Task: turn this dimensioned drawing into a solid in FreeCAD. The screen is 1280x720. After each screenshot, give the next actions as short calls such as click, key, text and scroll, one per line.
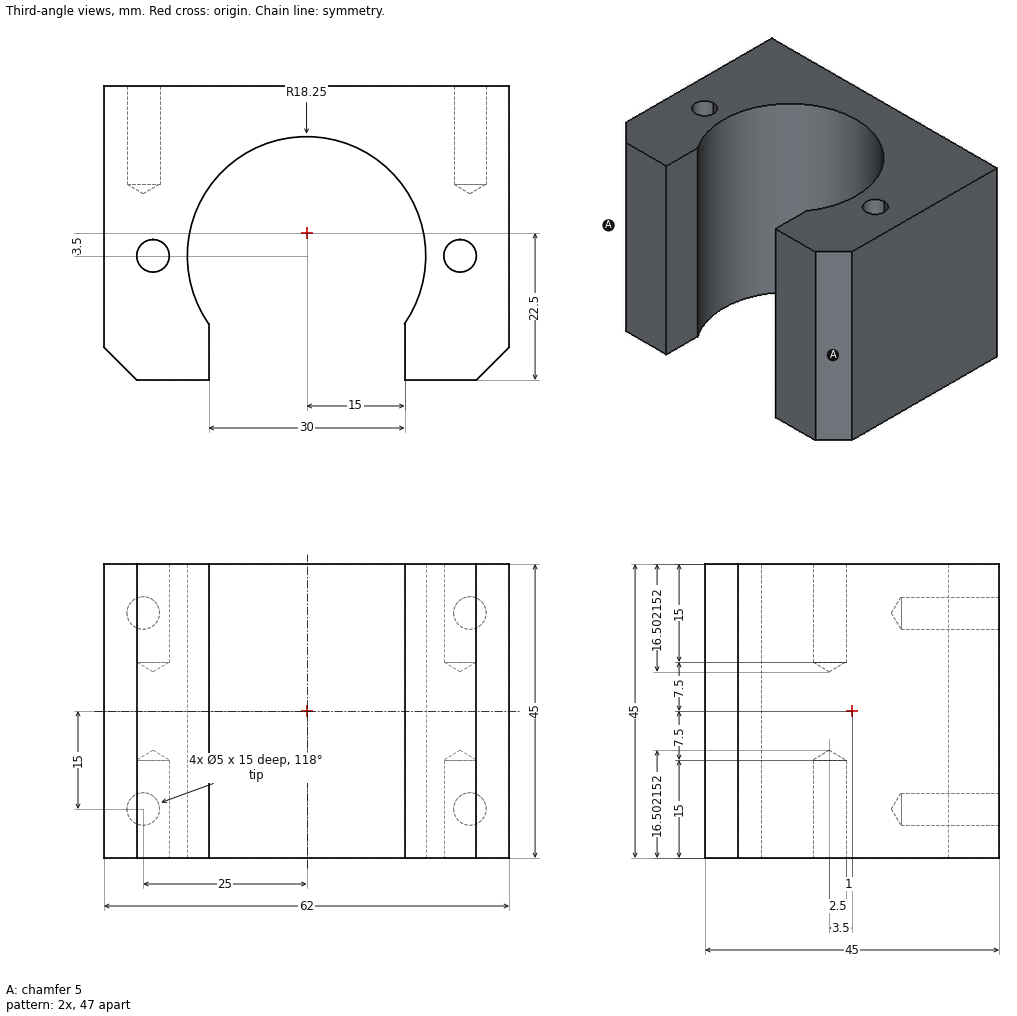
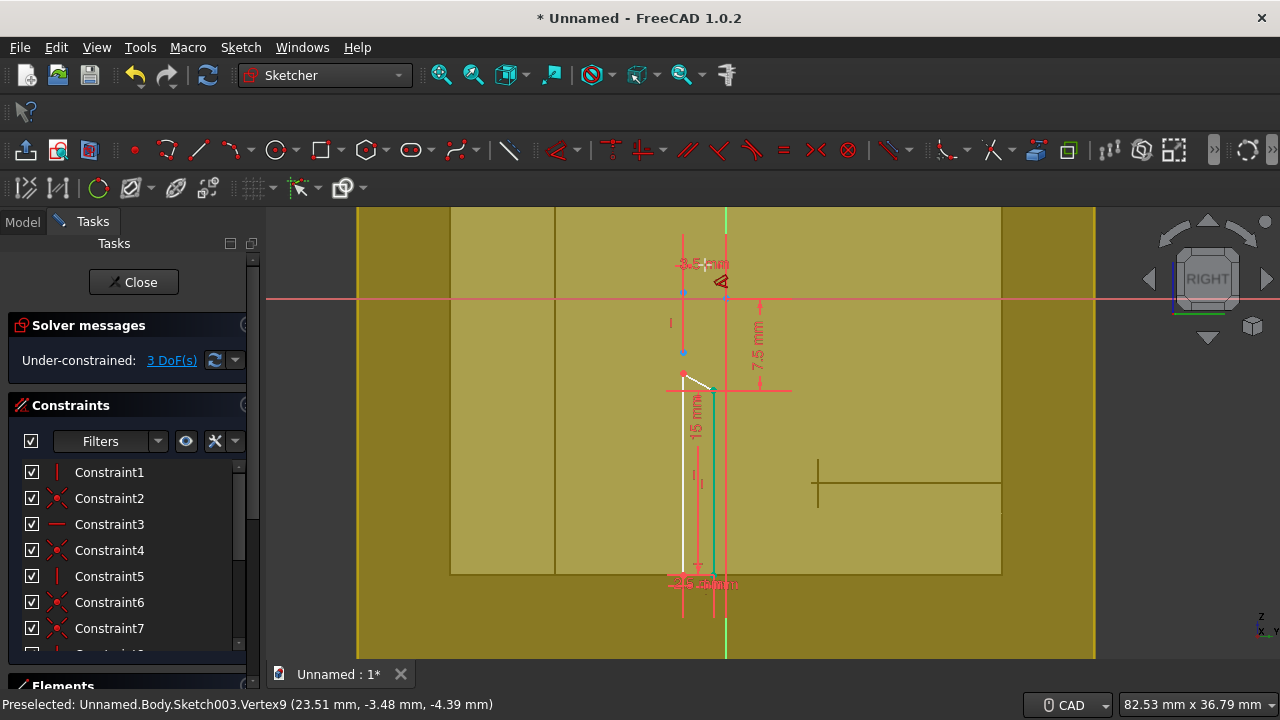
click(683, 434)
click(649, 475)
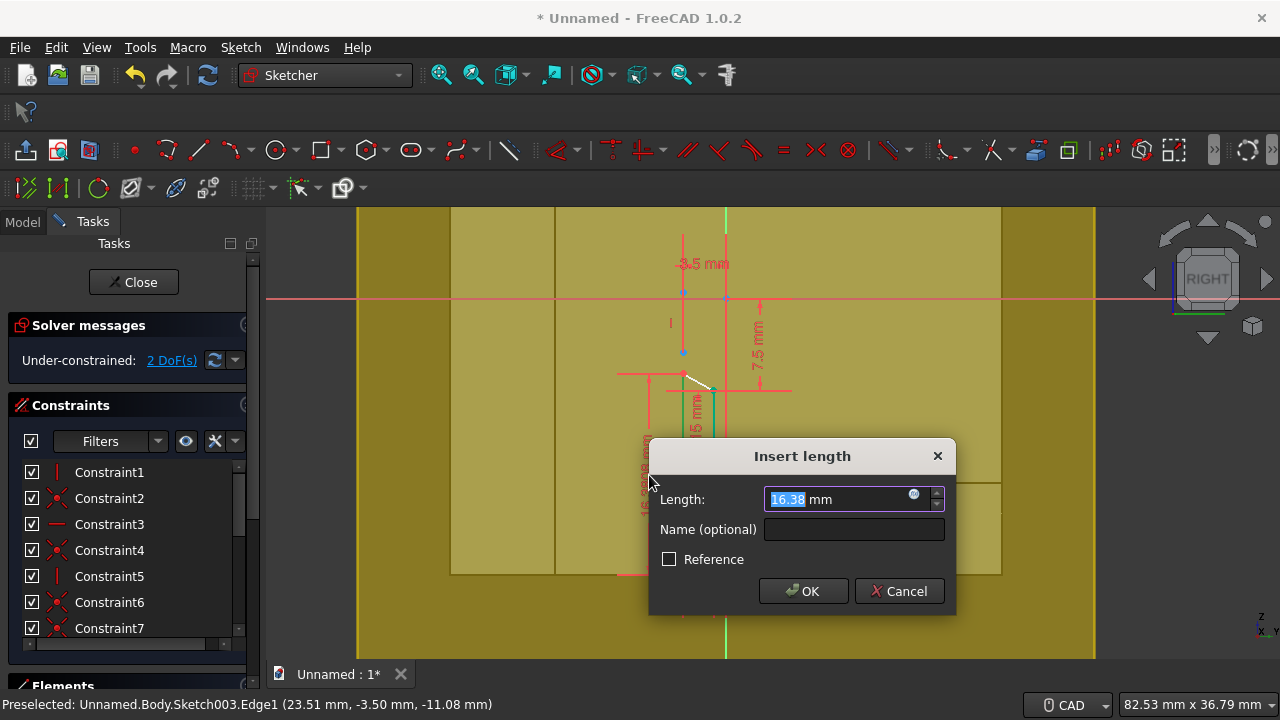
text(16.502152)
key(Return)
key(Escape)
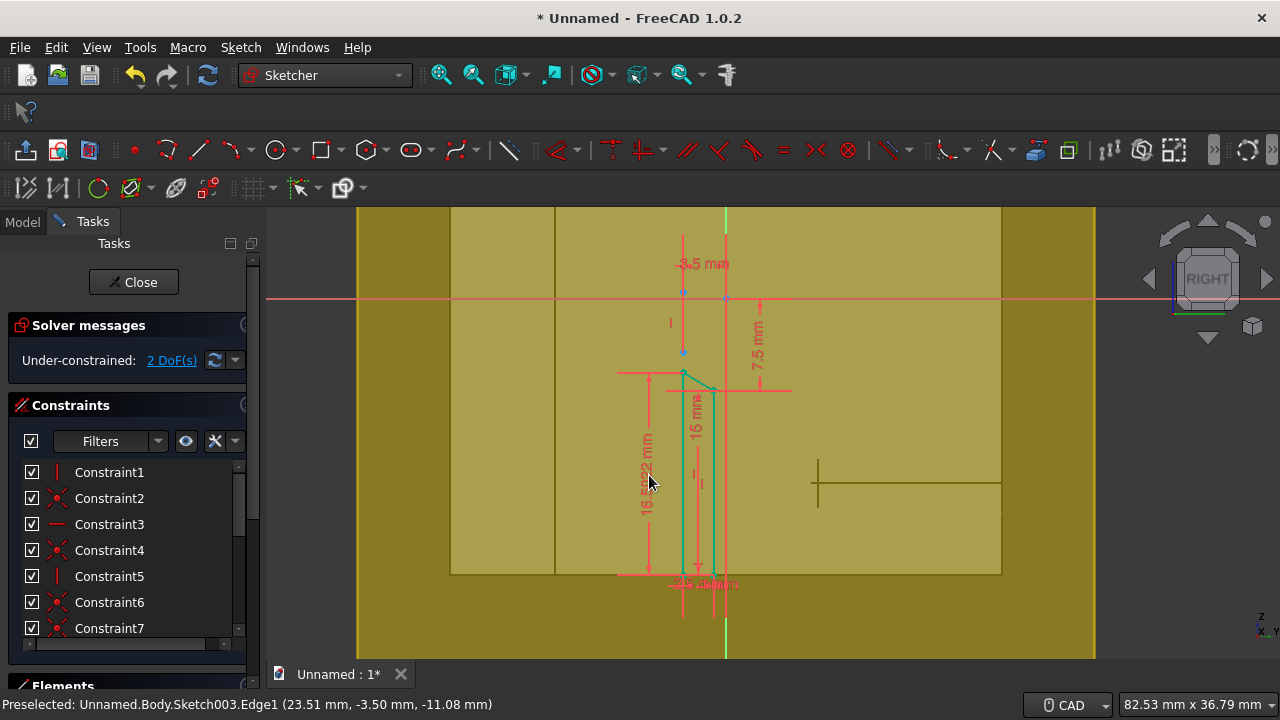
click(134, 282)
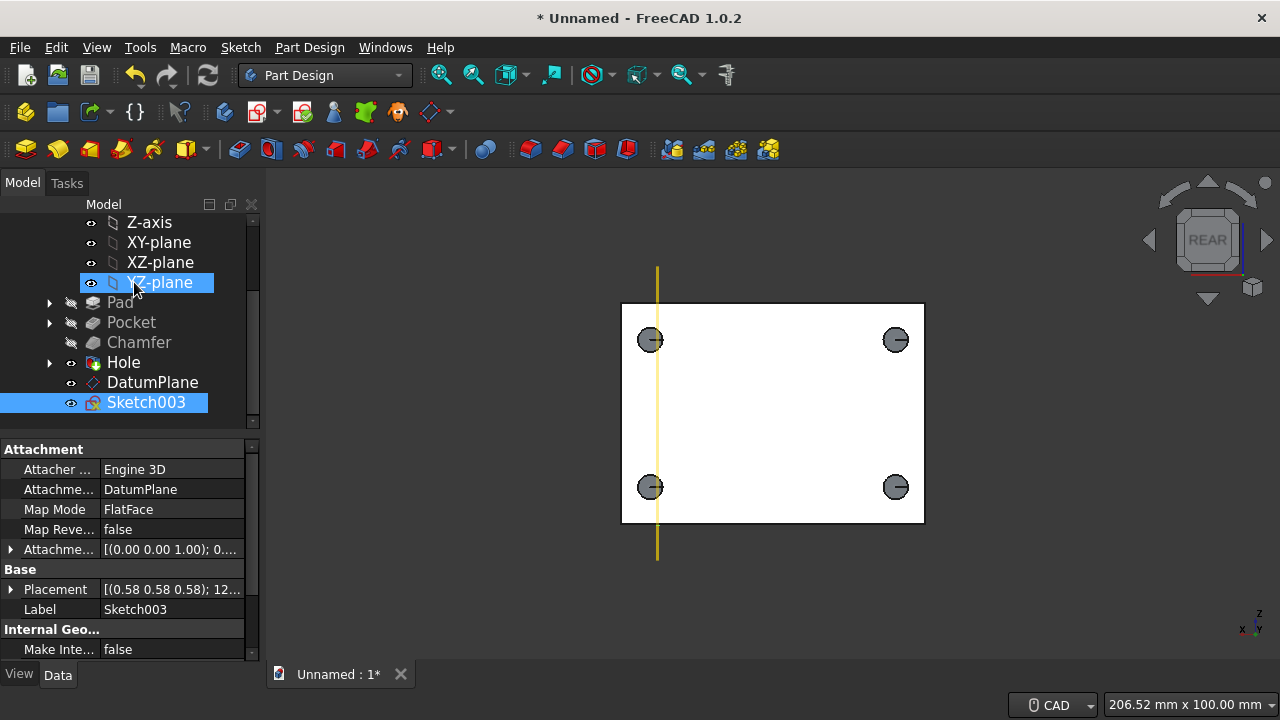
click(304, 150)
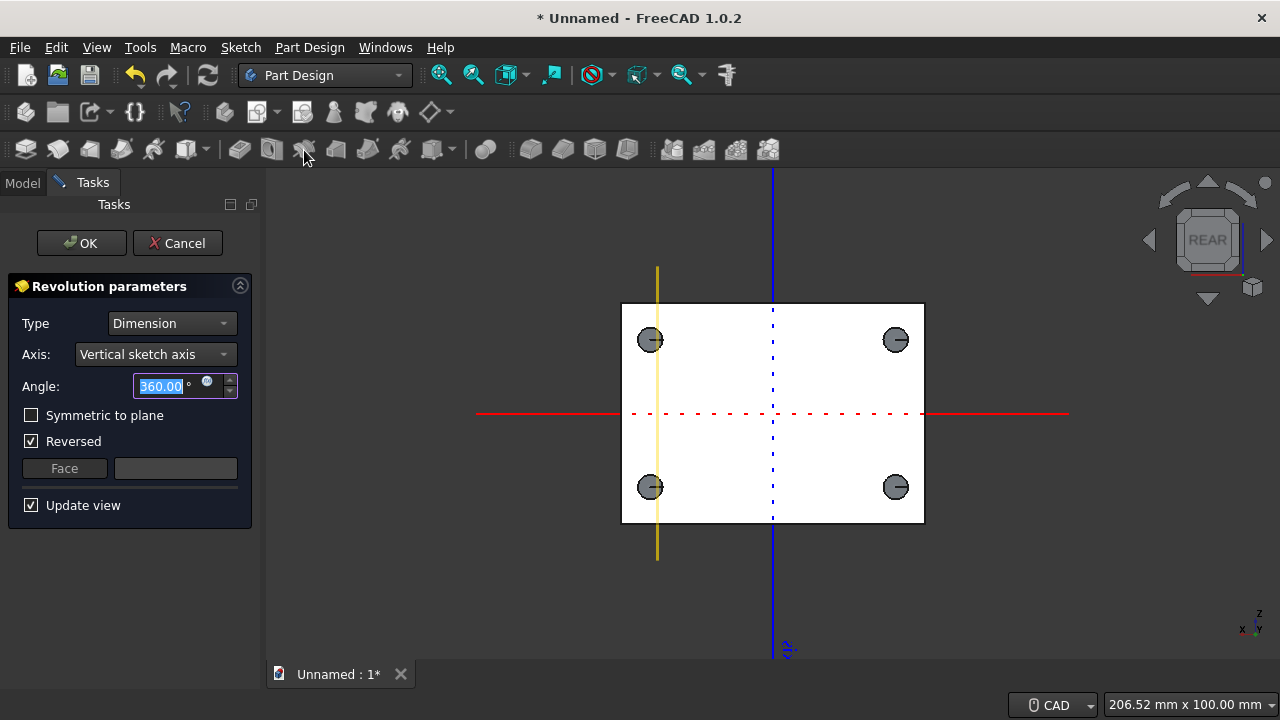
click(156, 354)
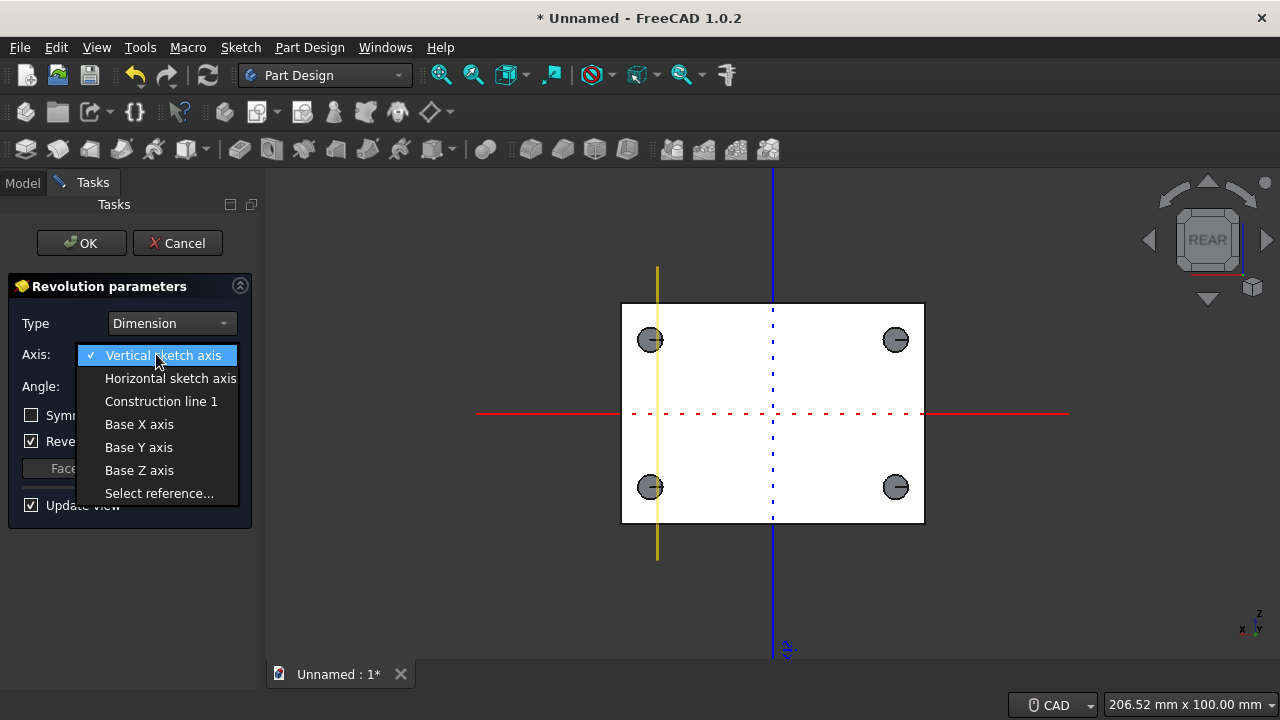
click(156, 402)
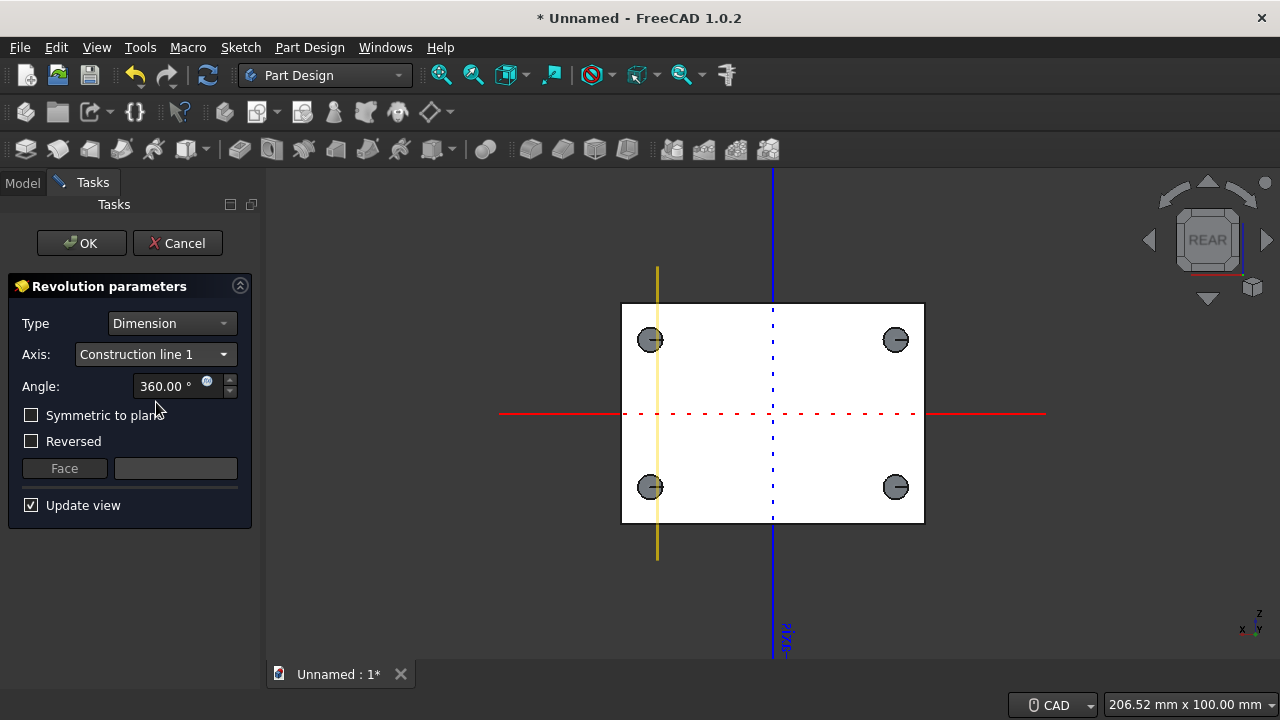
click(82, 243)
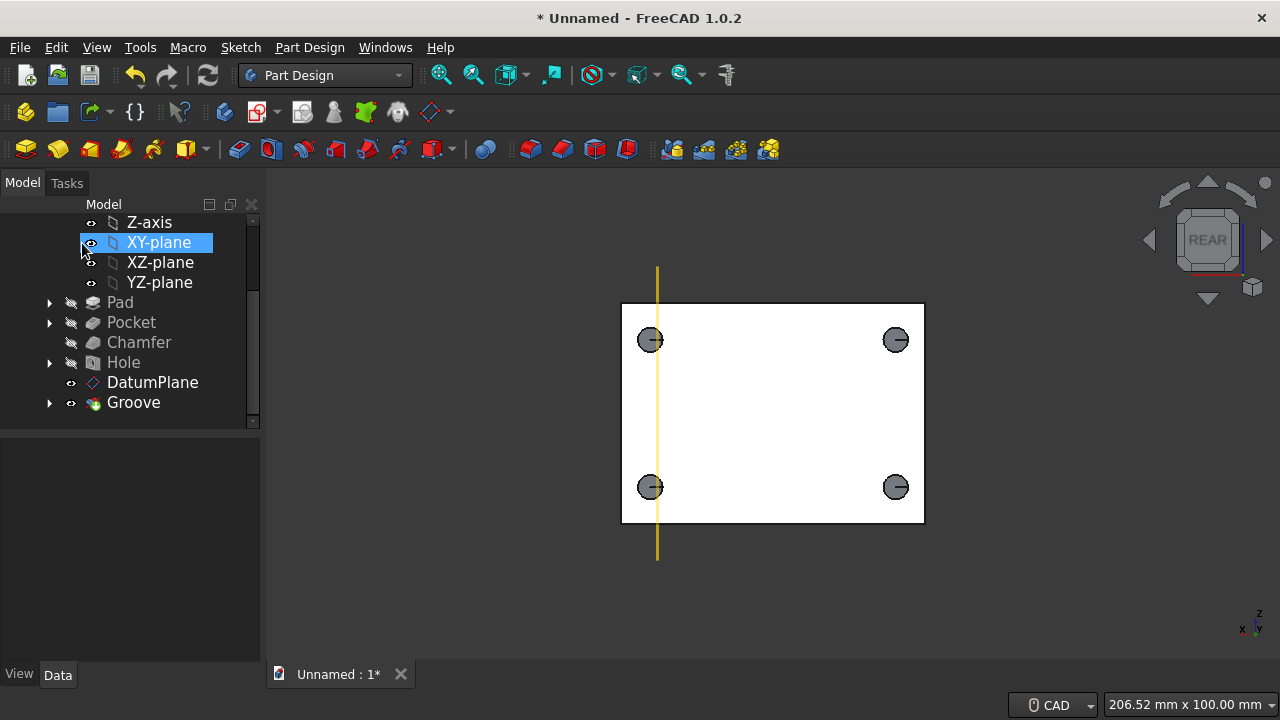
click(116, 383)
key(space)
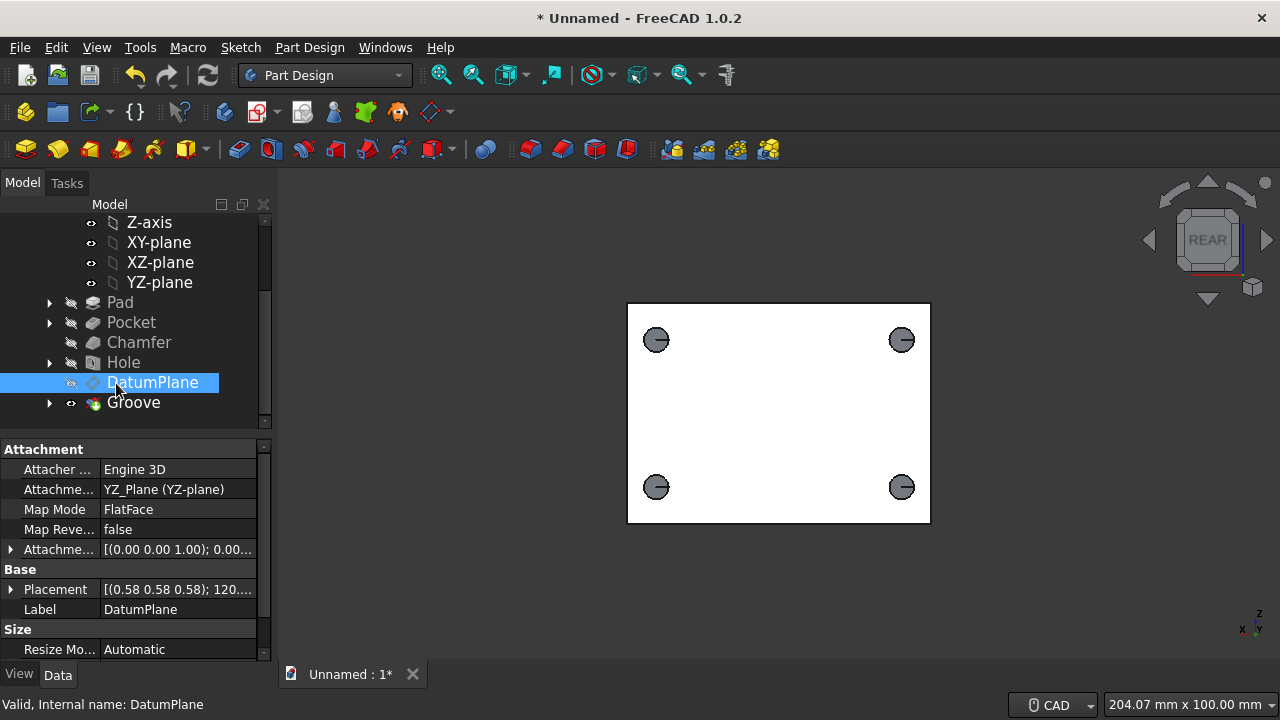
click(116, 403)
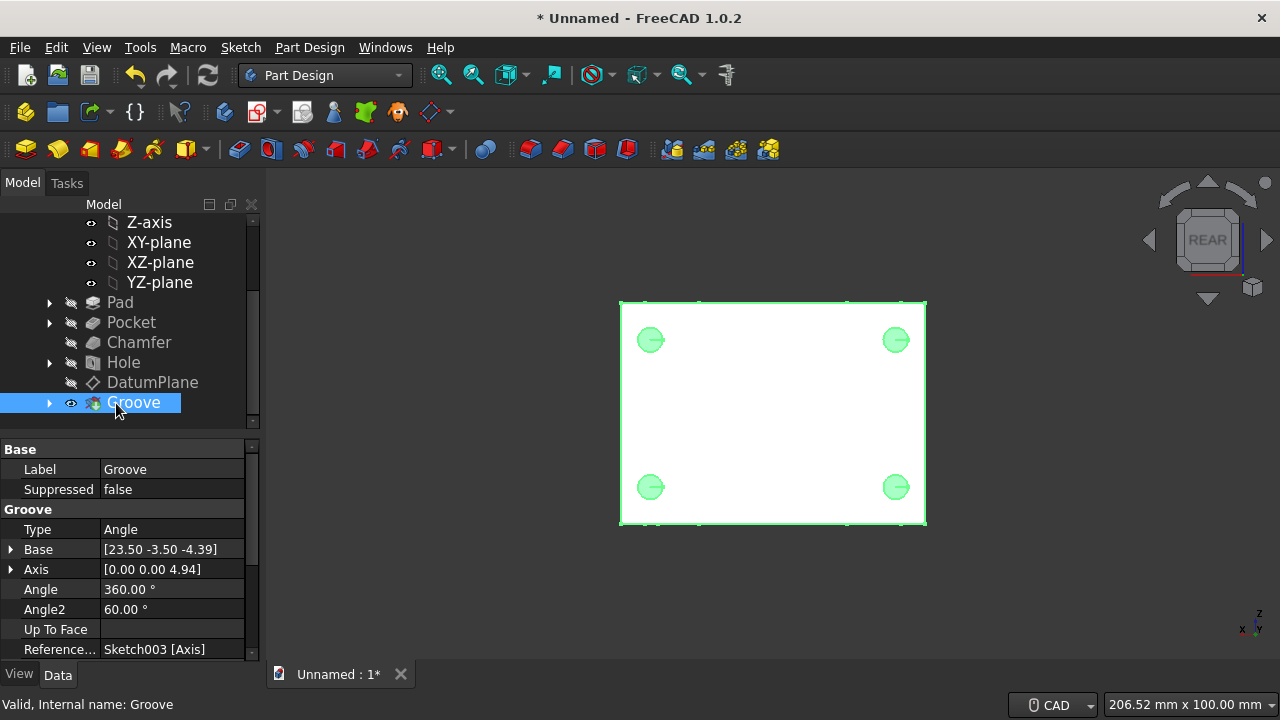
click(704, 150)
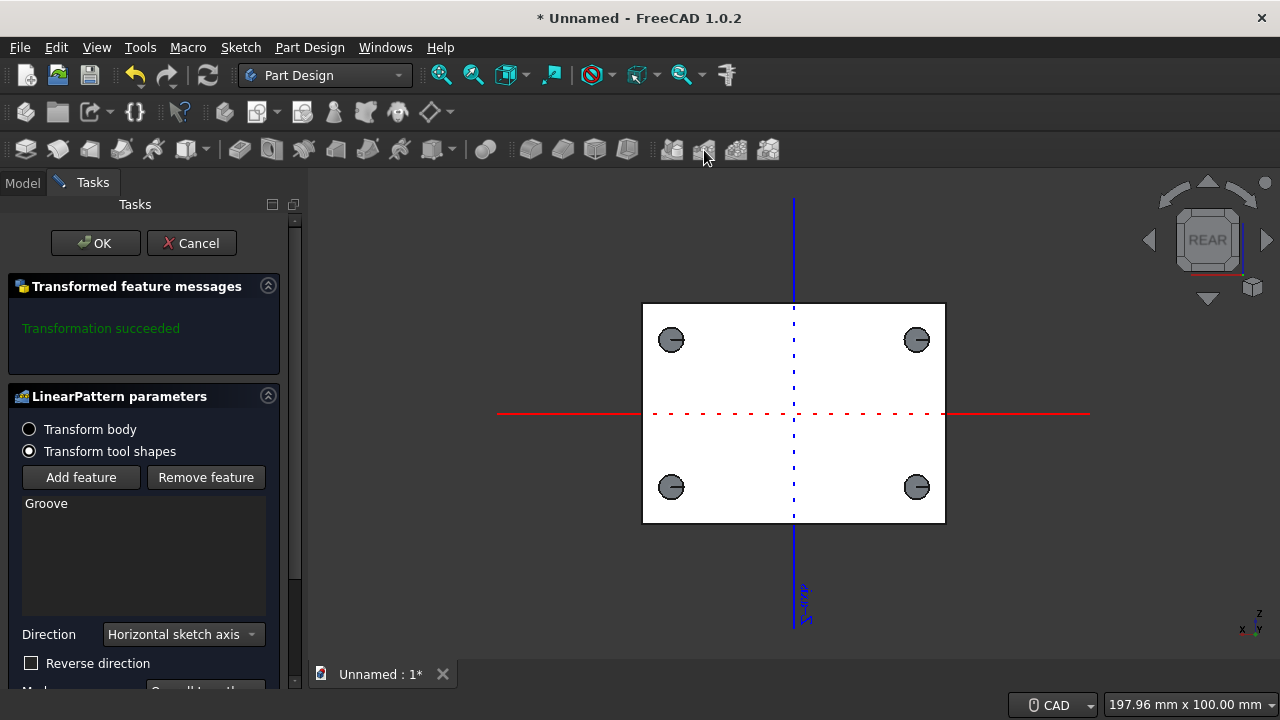
click(184, 634)